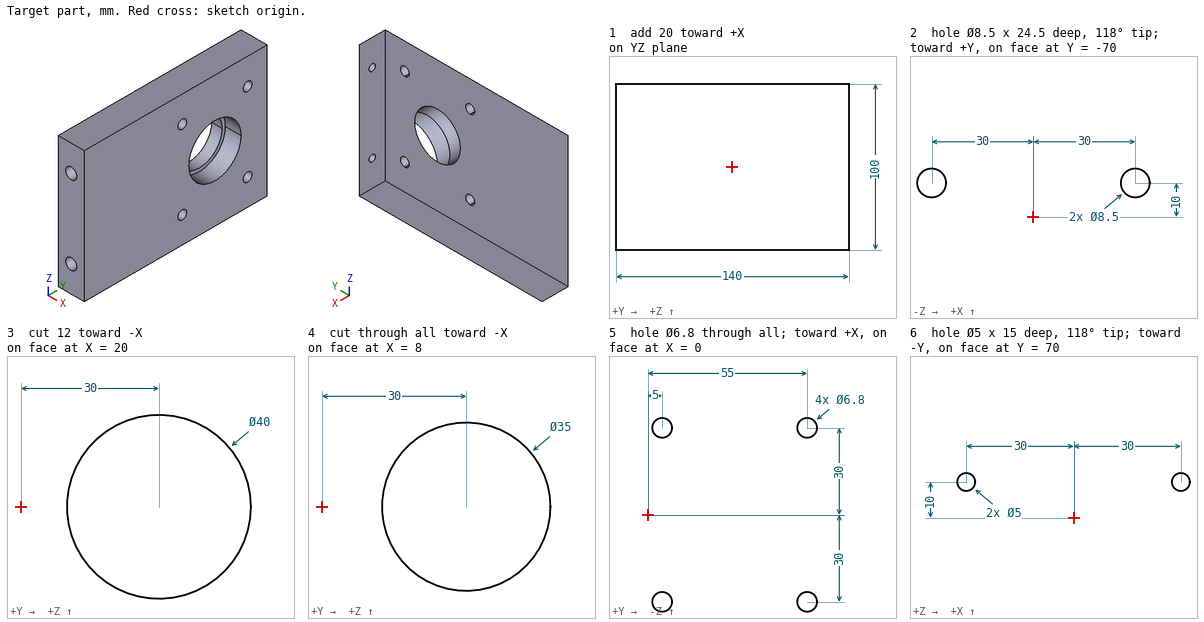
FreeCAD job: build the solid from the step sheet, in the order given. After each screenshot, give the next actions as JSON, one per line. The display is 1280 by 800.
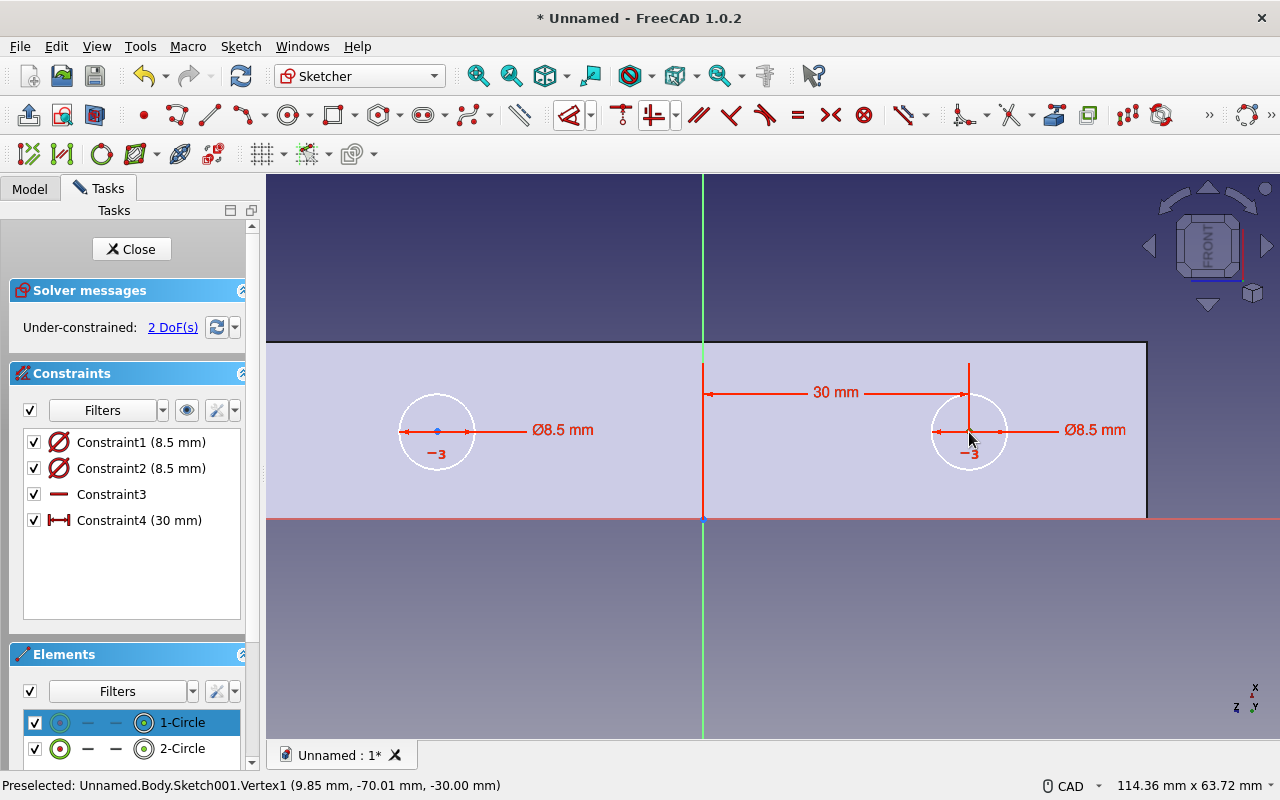
{"action": "left_click", "coordinate": [590, 116]}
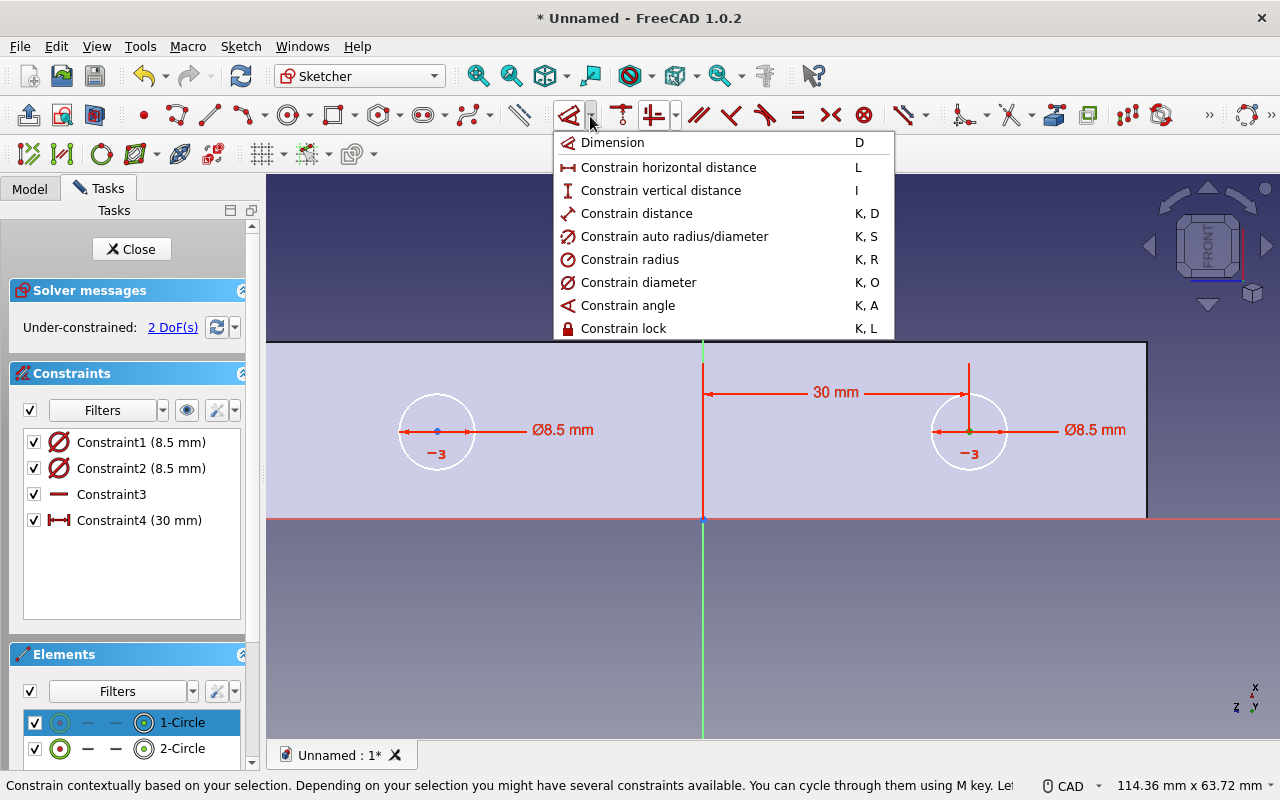
{"action": "left_click", "coordinate": [724, 190]}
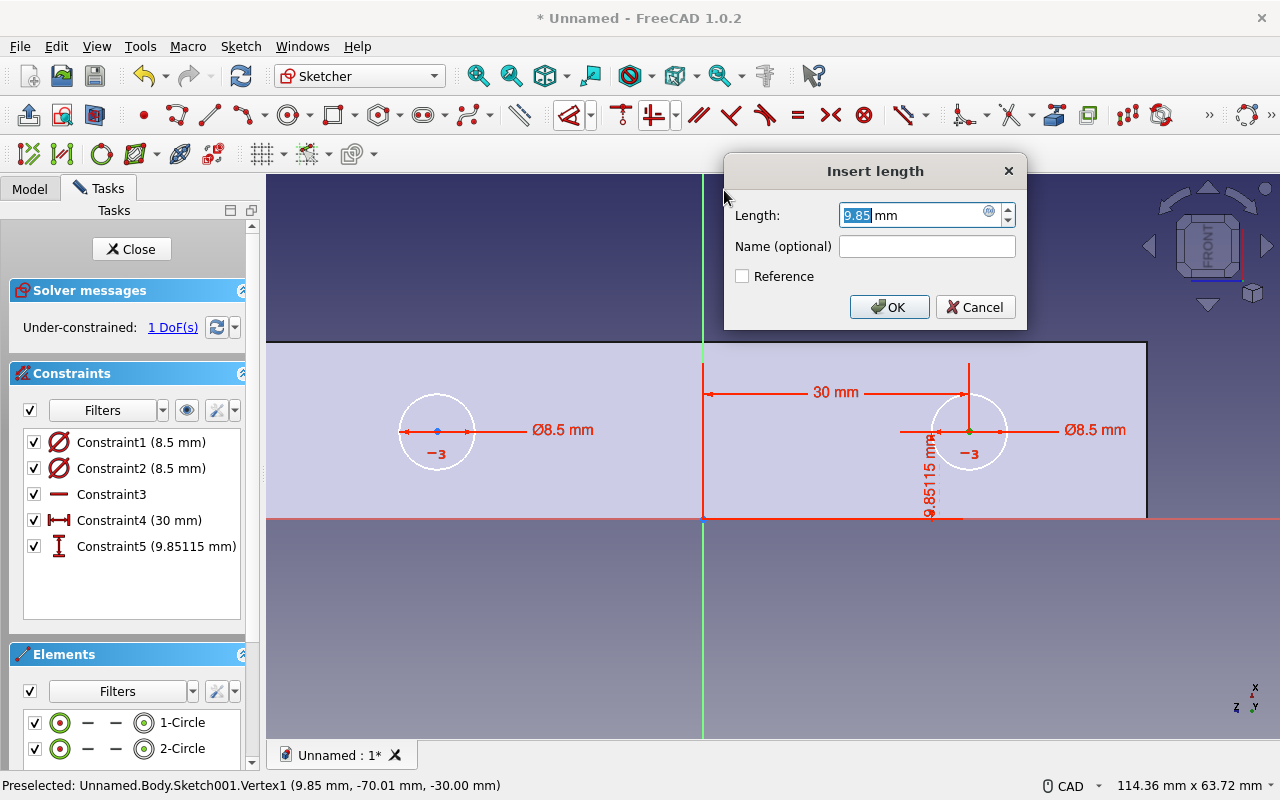
{"action": "type", "text": "10"}
{"action": "key", "text": "Return"}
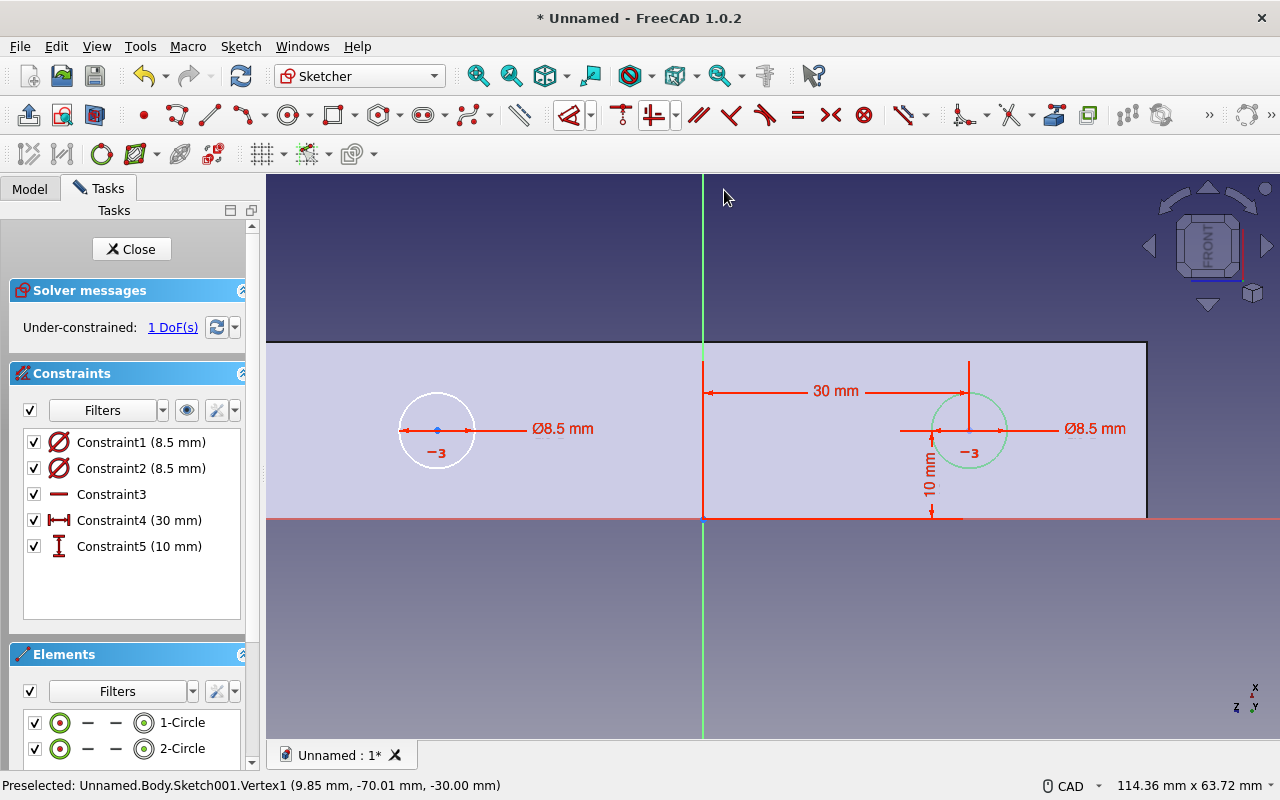
{"action": "left_click", "coordinate": [437, 431]}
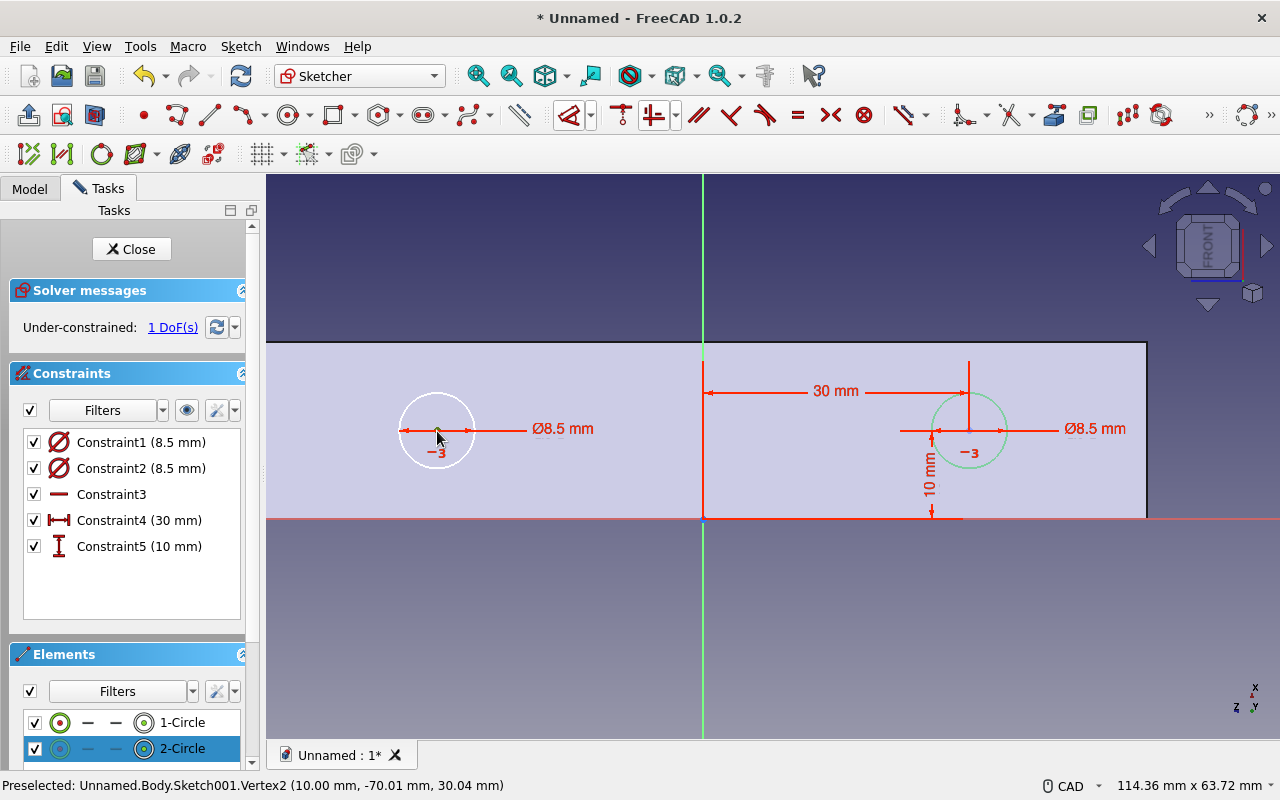
{"action": "key", "text": "l"}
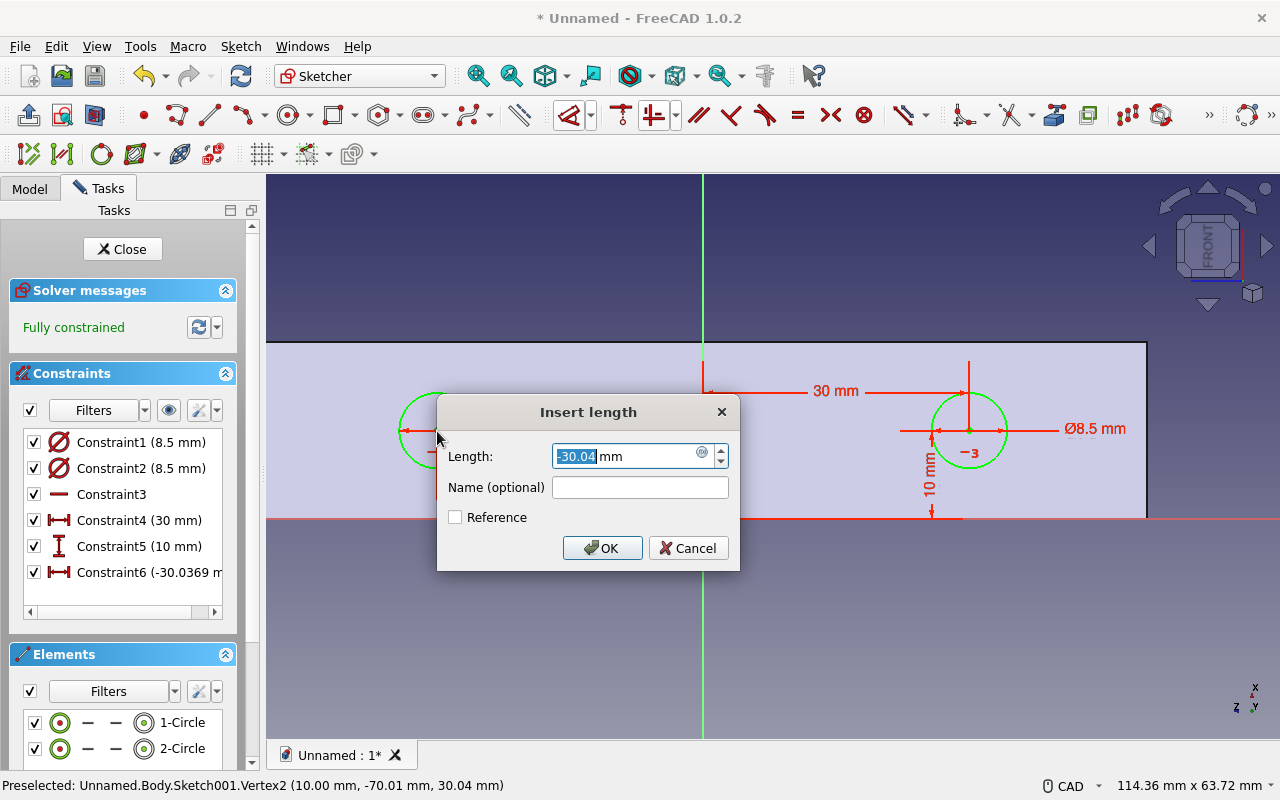
{"action": "type", "text": "-30"}
{"action": "key", "text": "Return"}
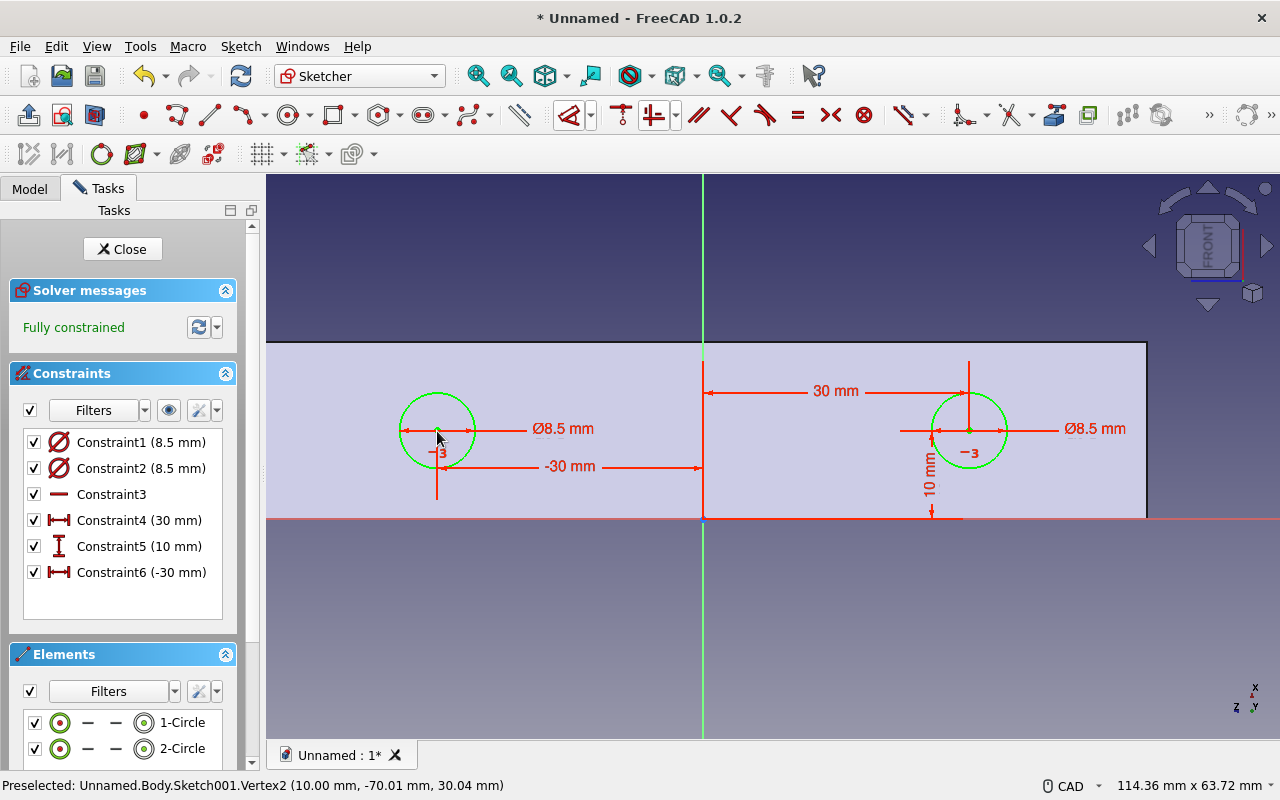
{"action": "left_click", "coordinate": [123, 249]}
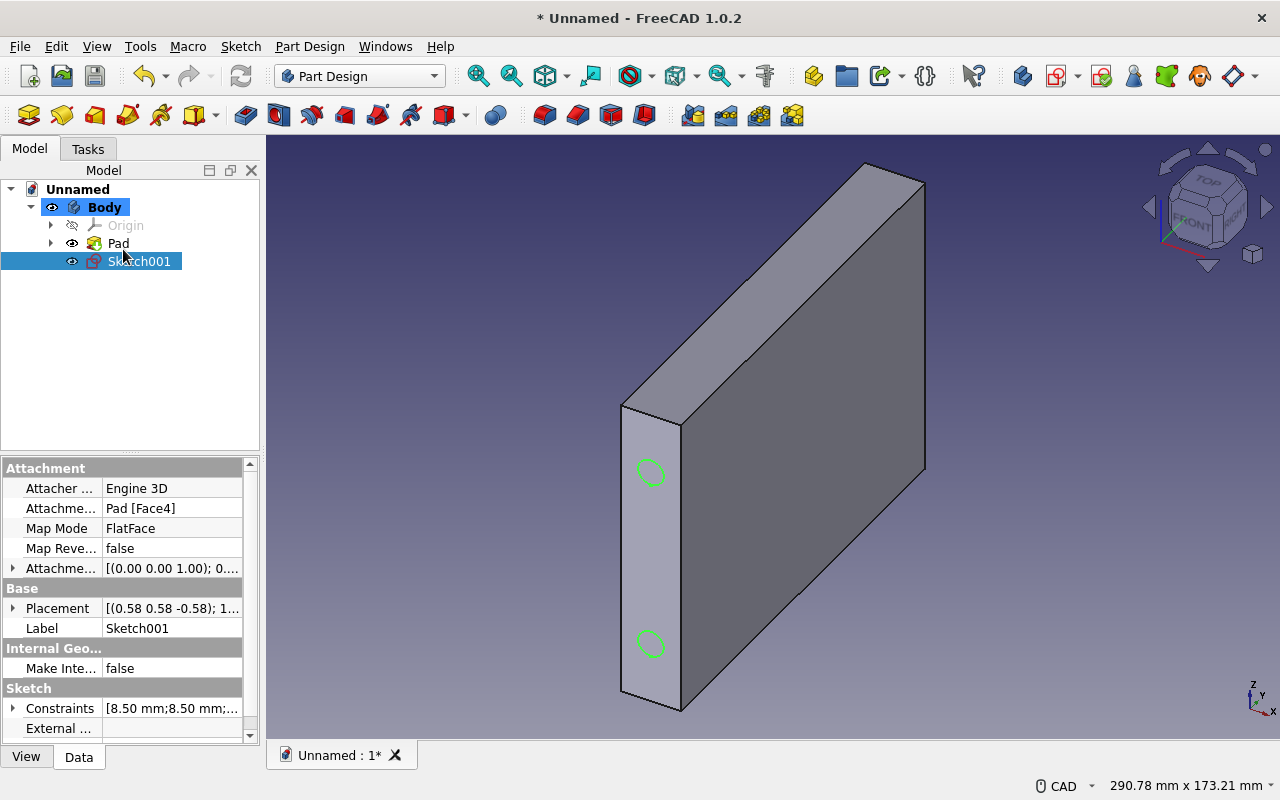
{"action": "left_click", "coordinate": [279, 116]}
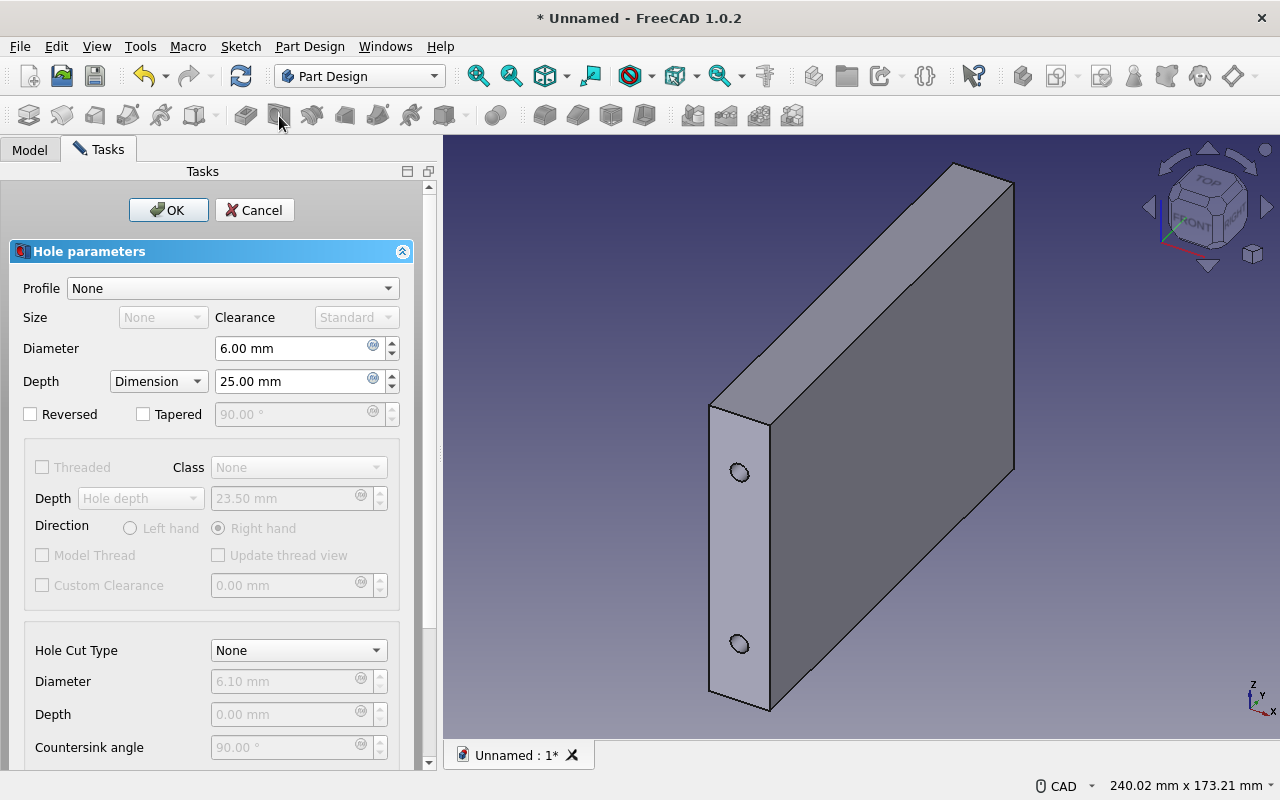
{"action": "triple_click", "coordinate": [300, 348]}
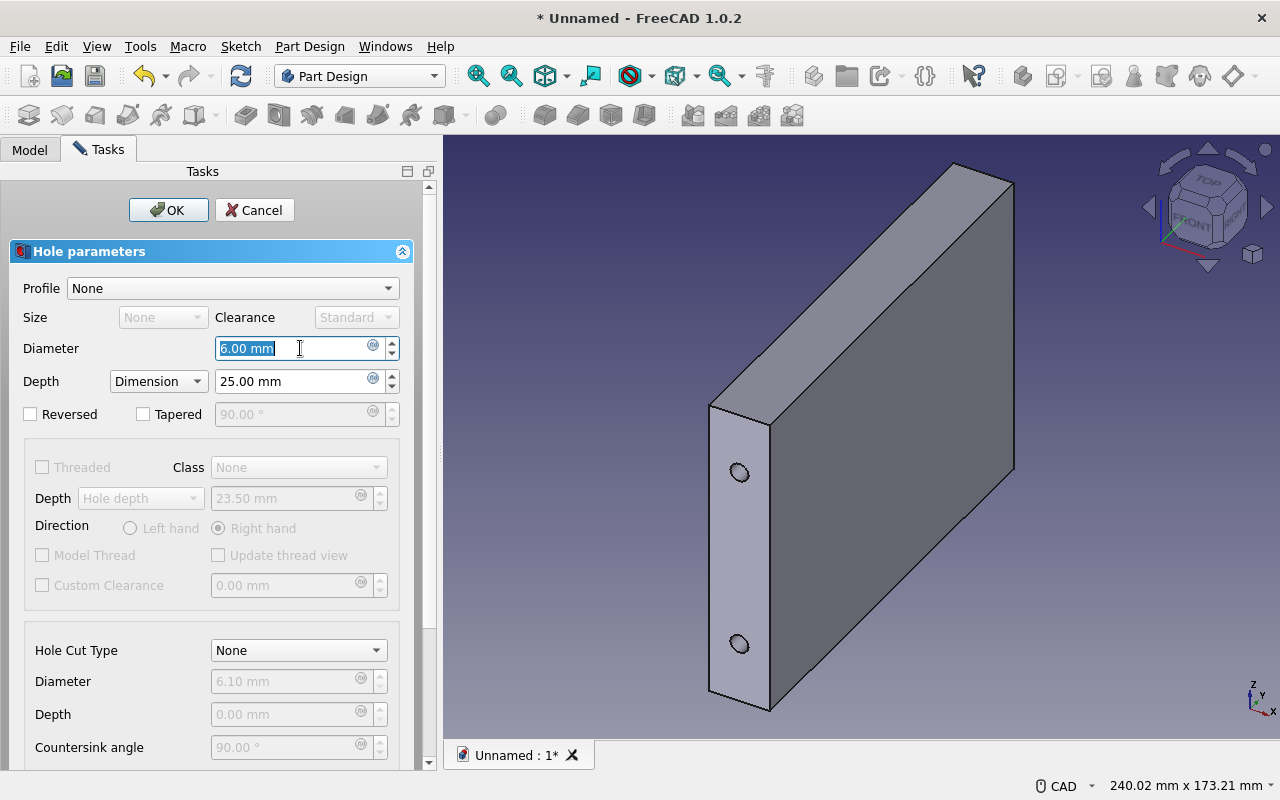
{"action": "type", "text": "8.5"}
{"action": "key", "text": "Tab"}